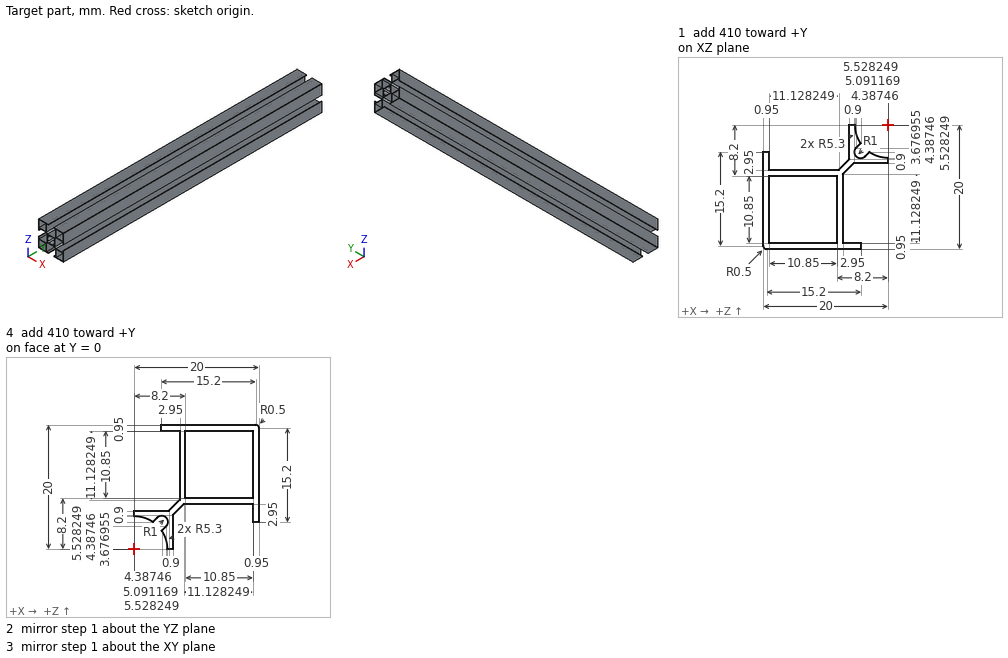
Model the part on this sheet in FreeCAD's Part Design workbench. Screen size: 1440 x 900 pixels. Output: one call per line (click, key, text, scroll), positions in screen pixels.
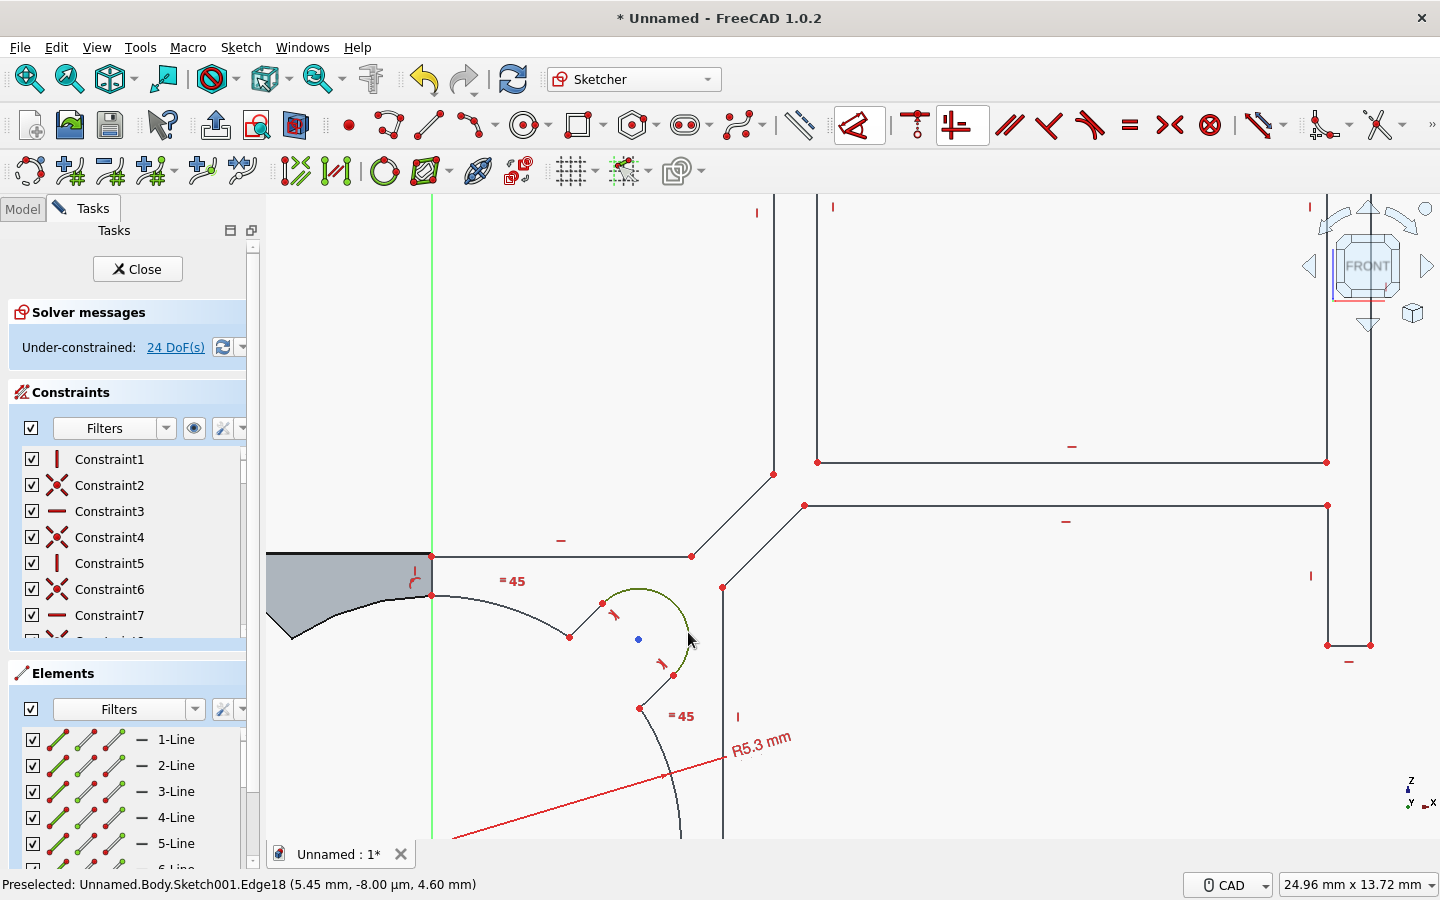
key(k)
key(r)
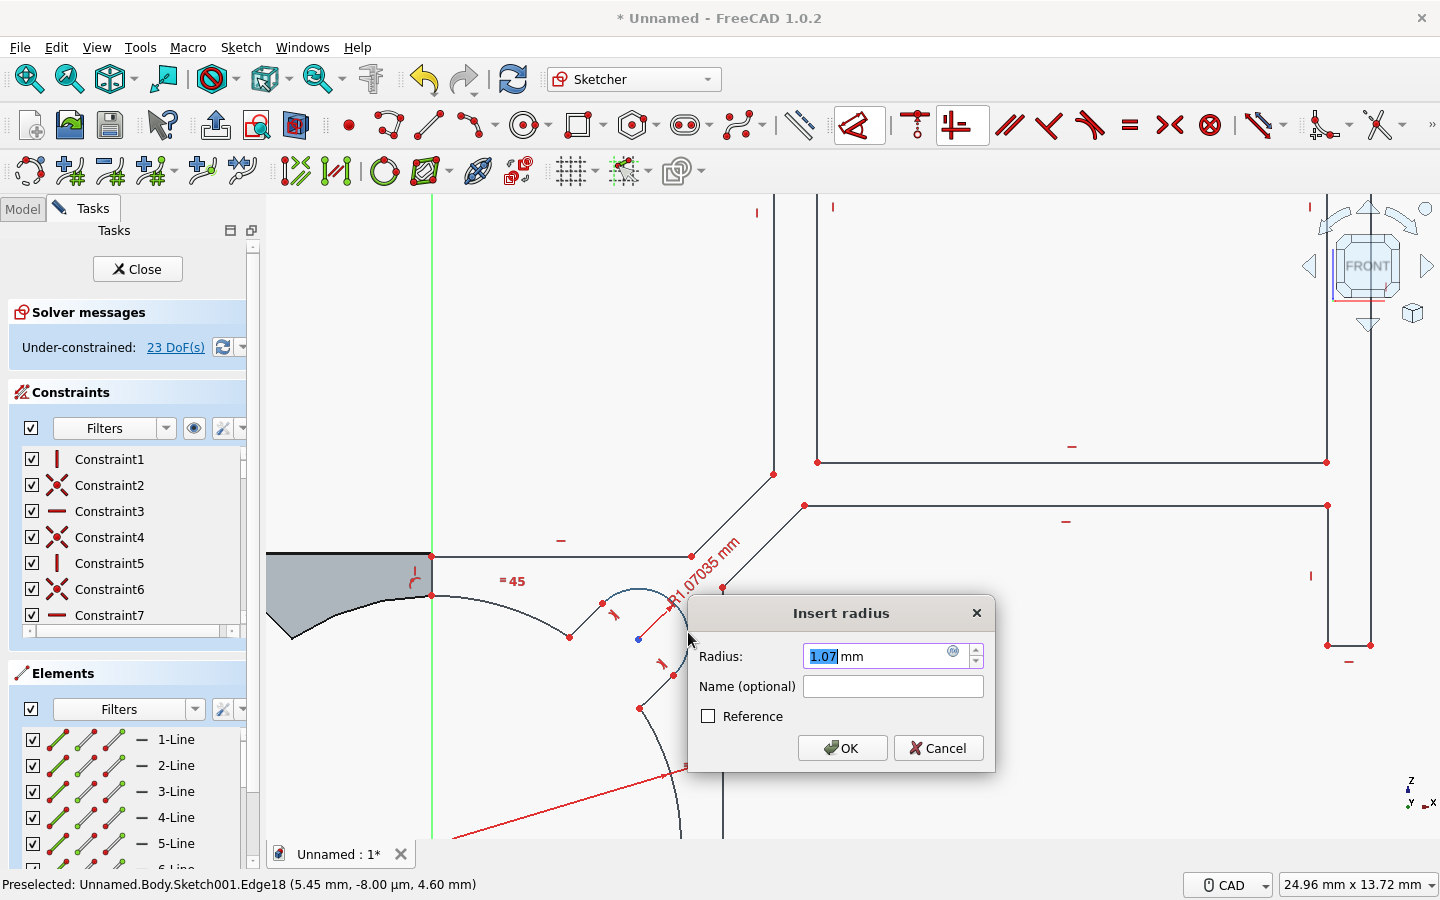
text(1)
key(Return)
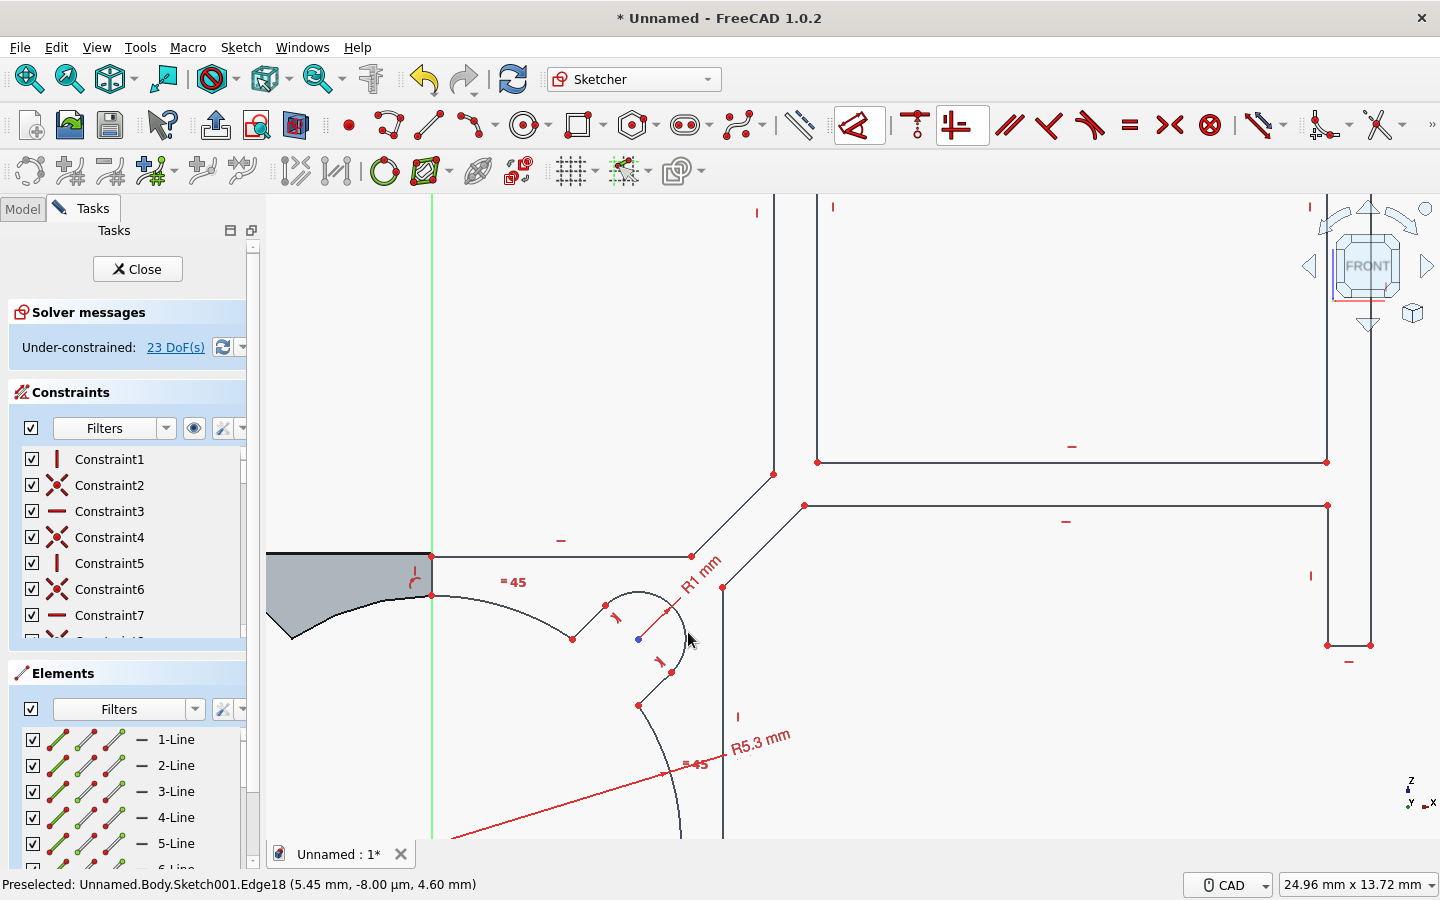
scroll(689, 632, down, 4)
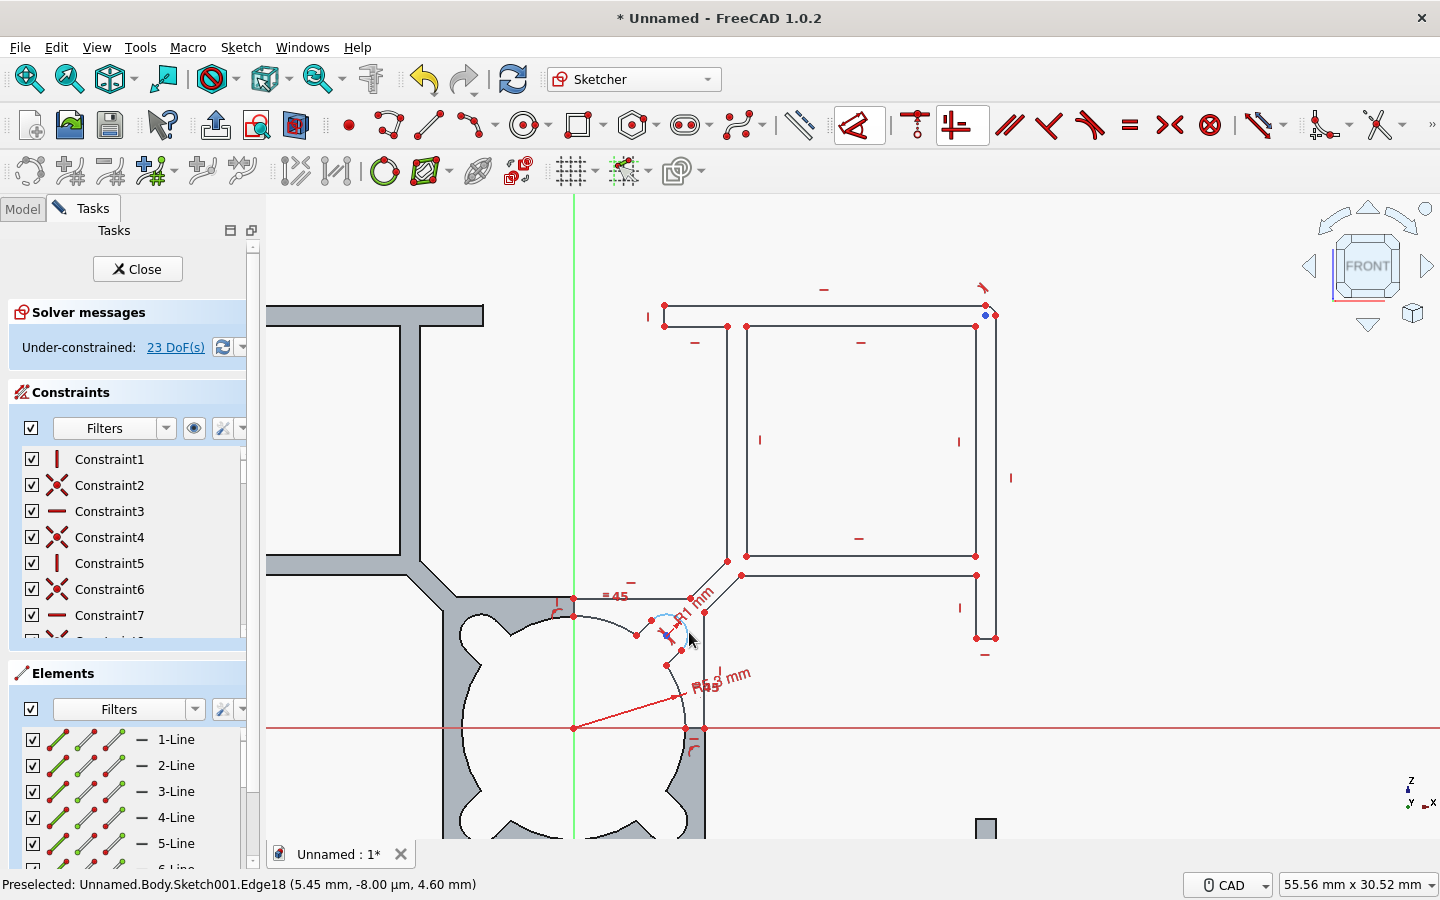
scroll(994, 311, up, 7)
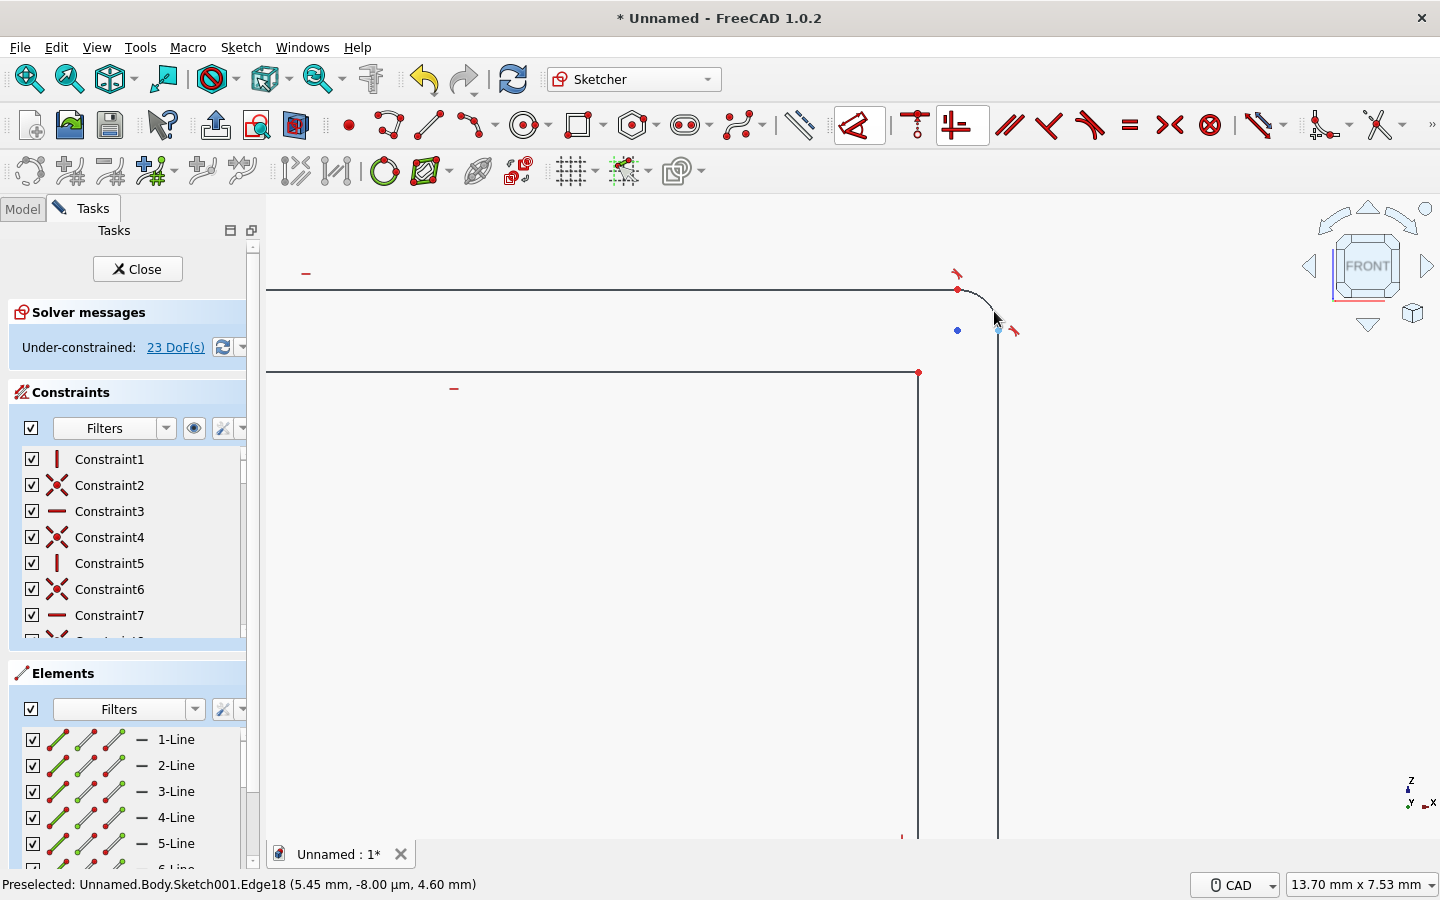
click(994, 312)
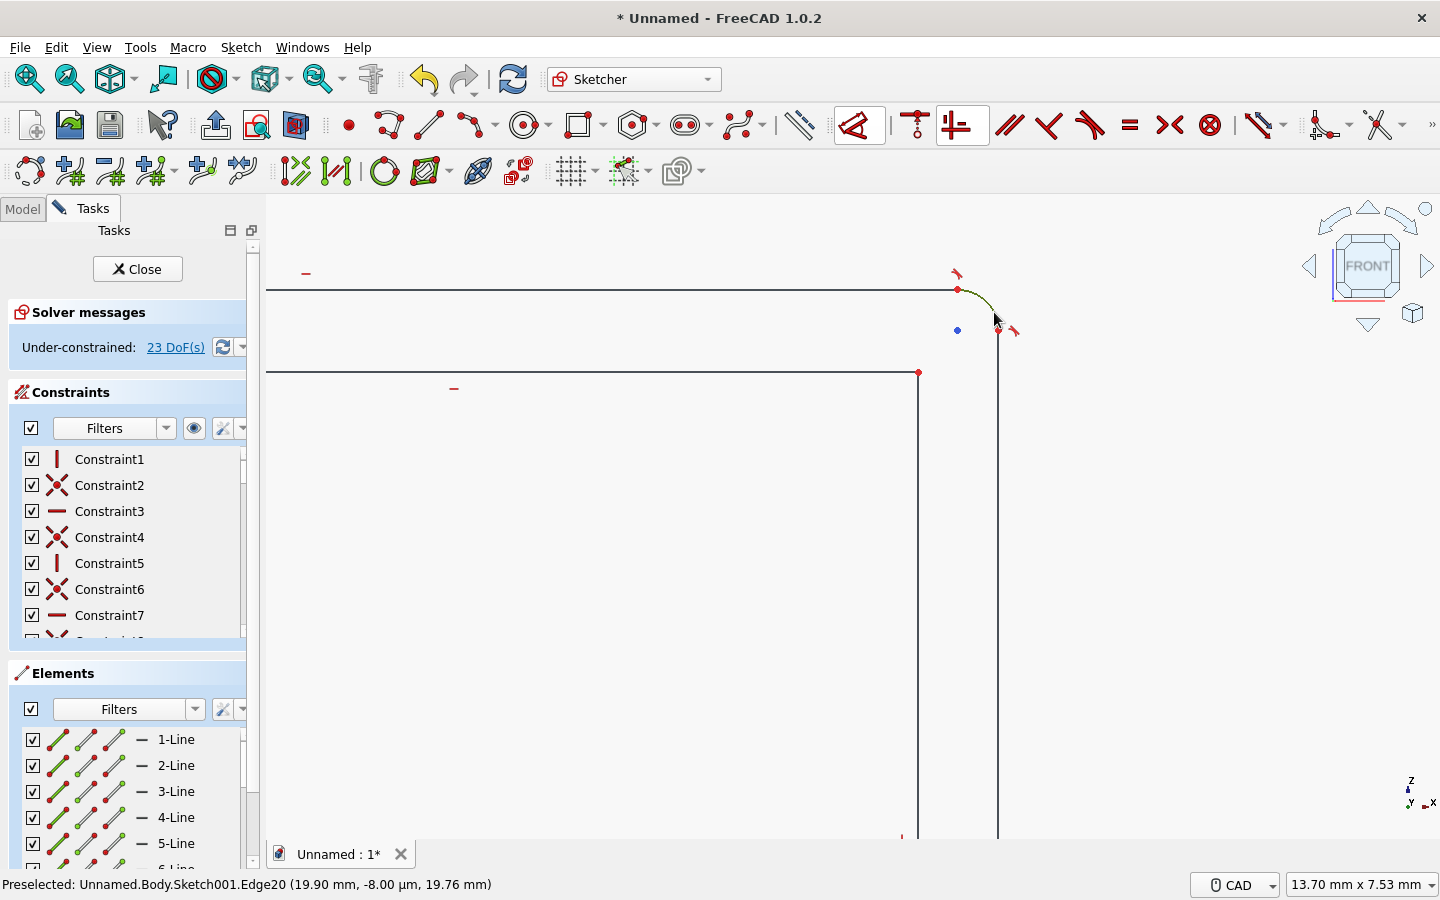
click(880, 126)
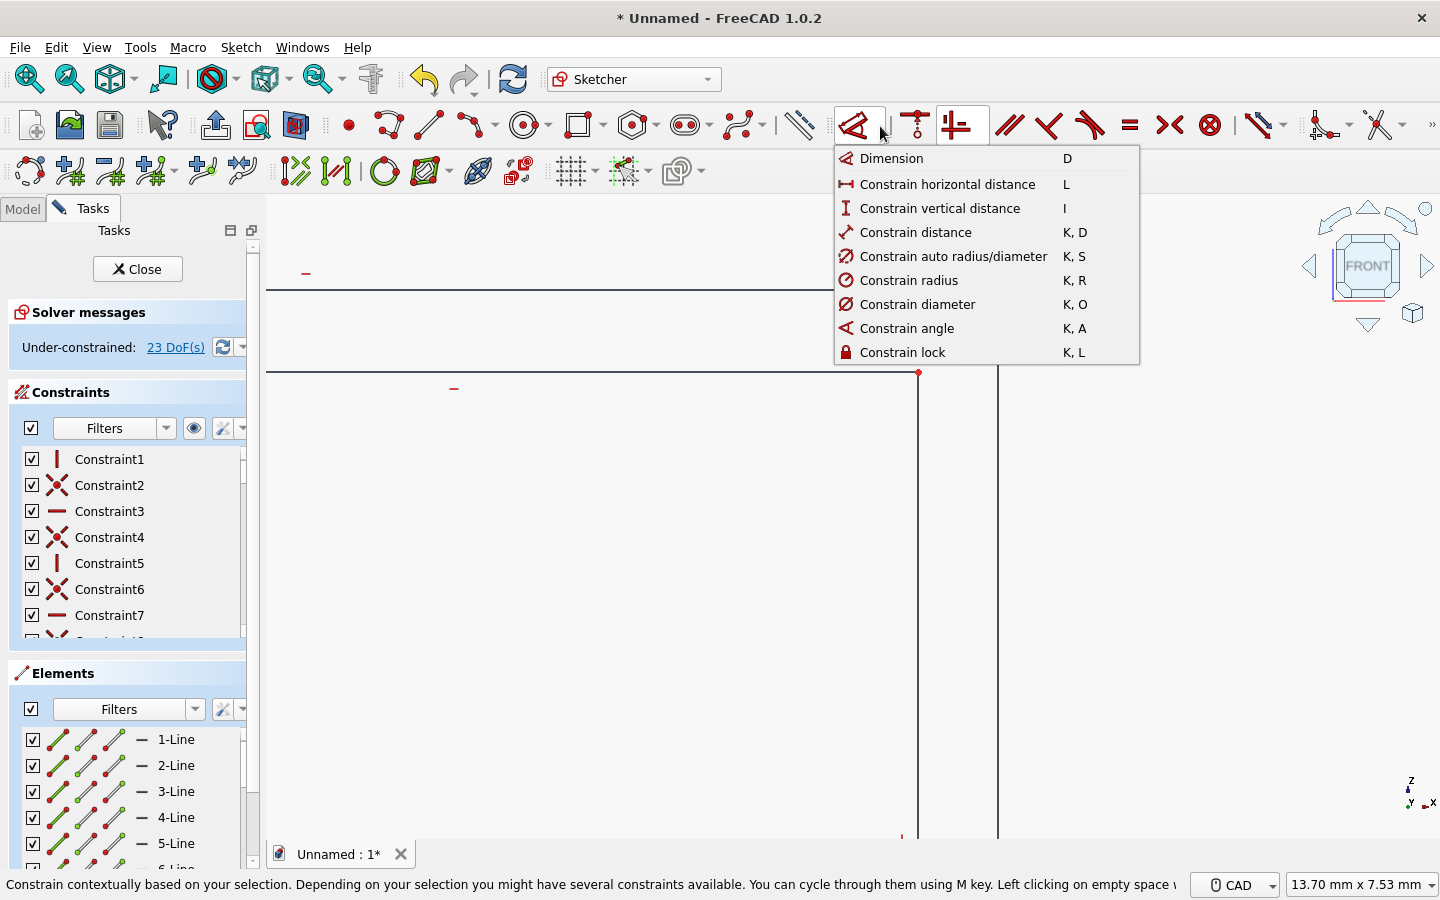
click(987, 280)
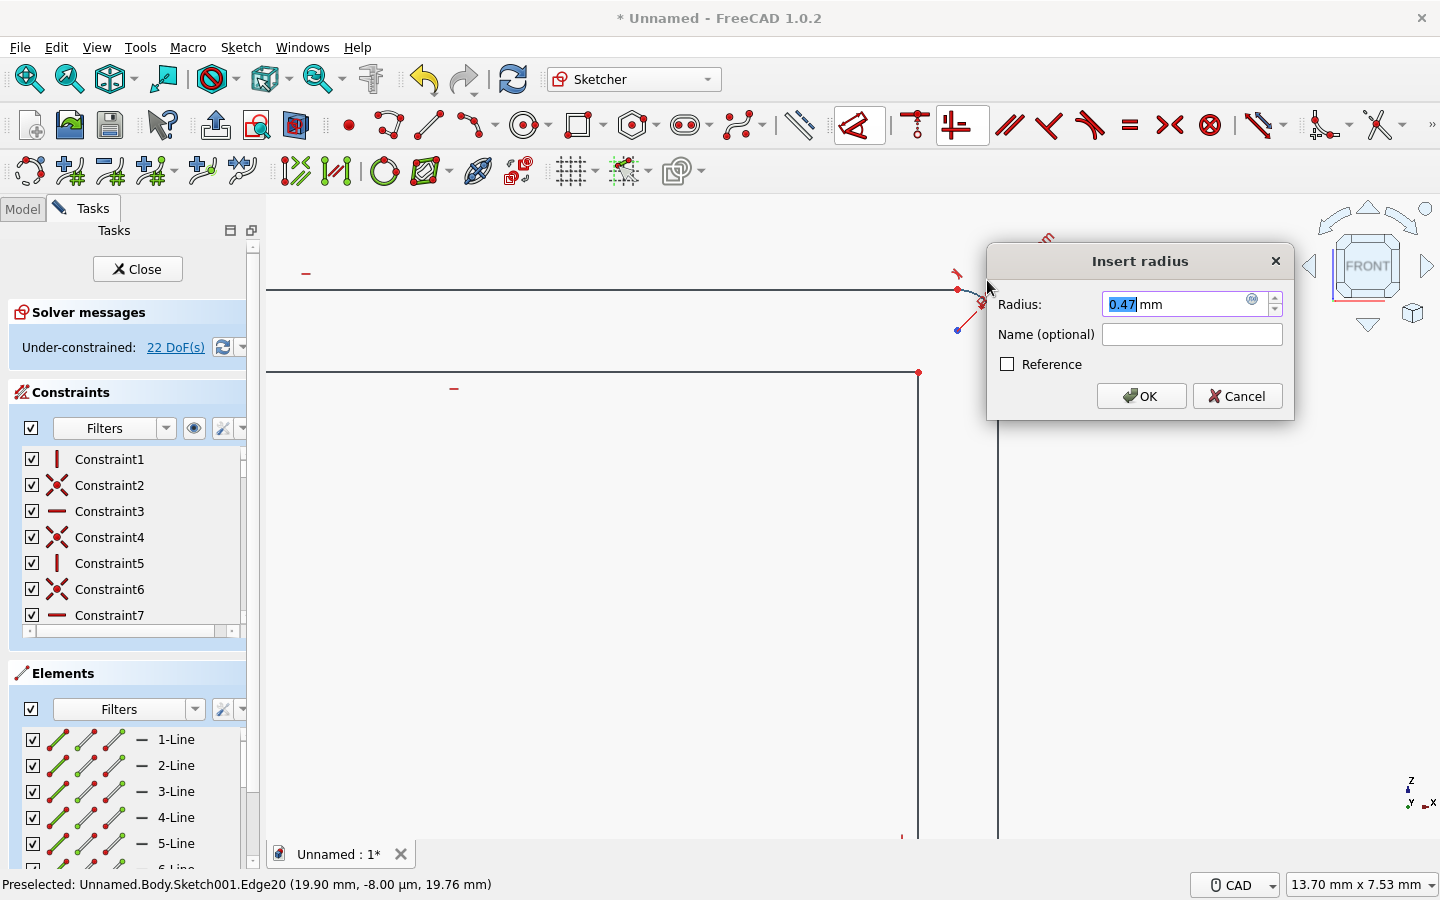
text(0.5)
key(Return)